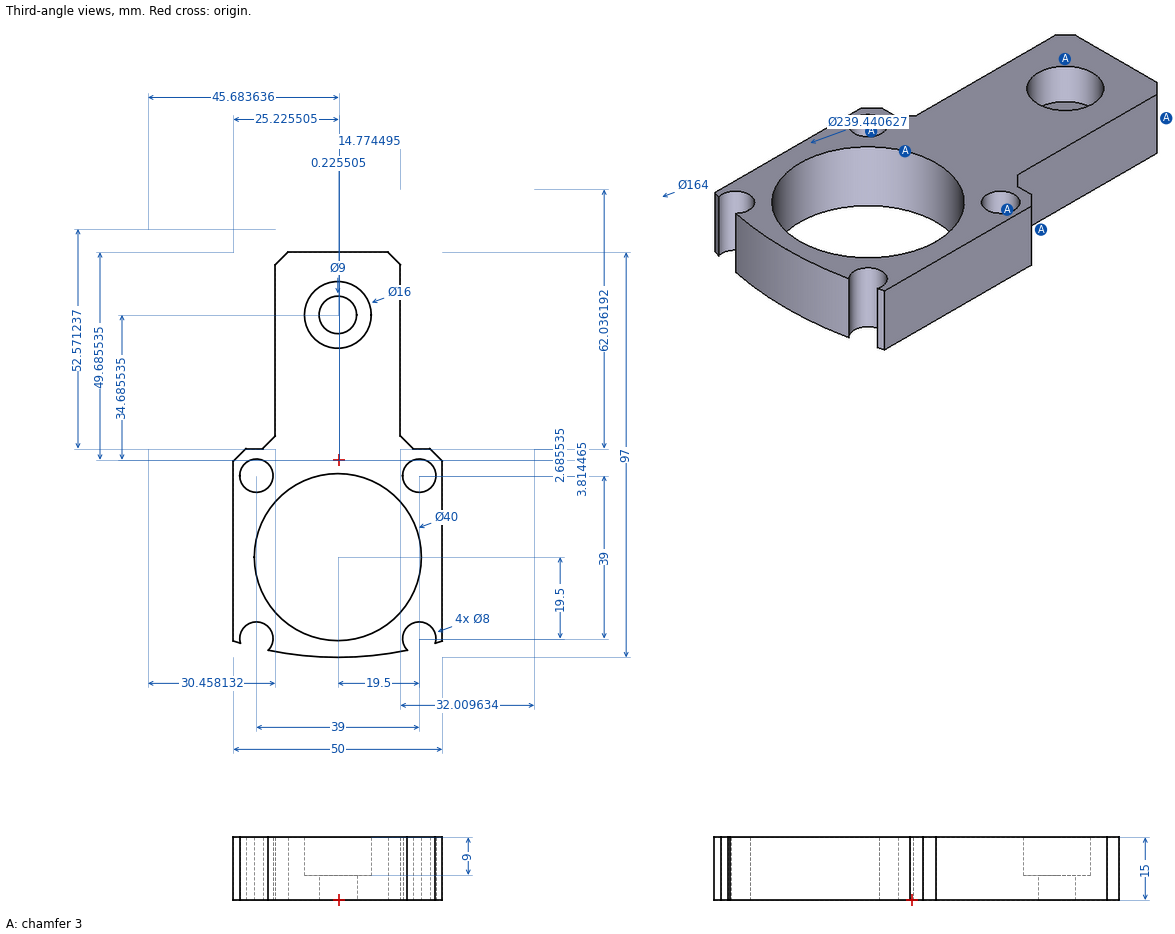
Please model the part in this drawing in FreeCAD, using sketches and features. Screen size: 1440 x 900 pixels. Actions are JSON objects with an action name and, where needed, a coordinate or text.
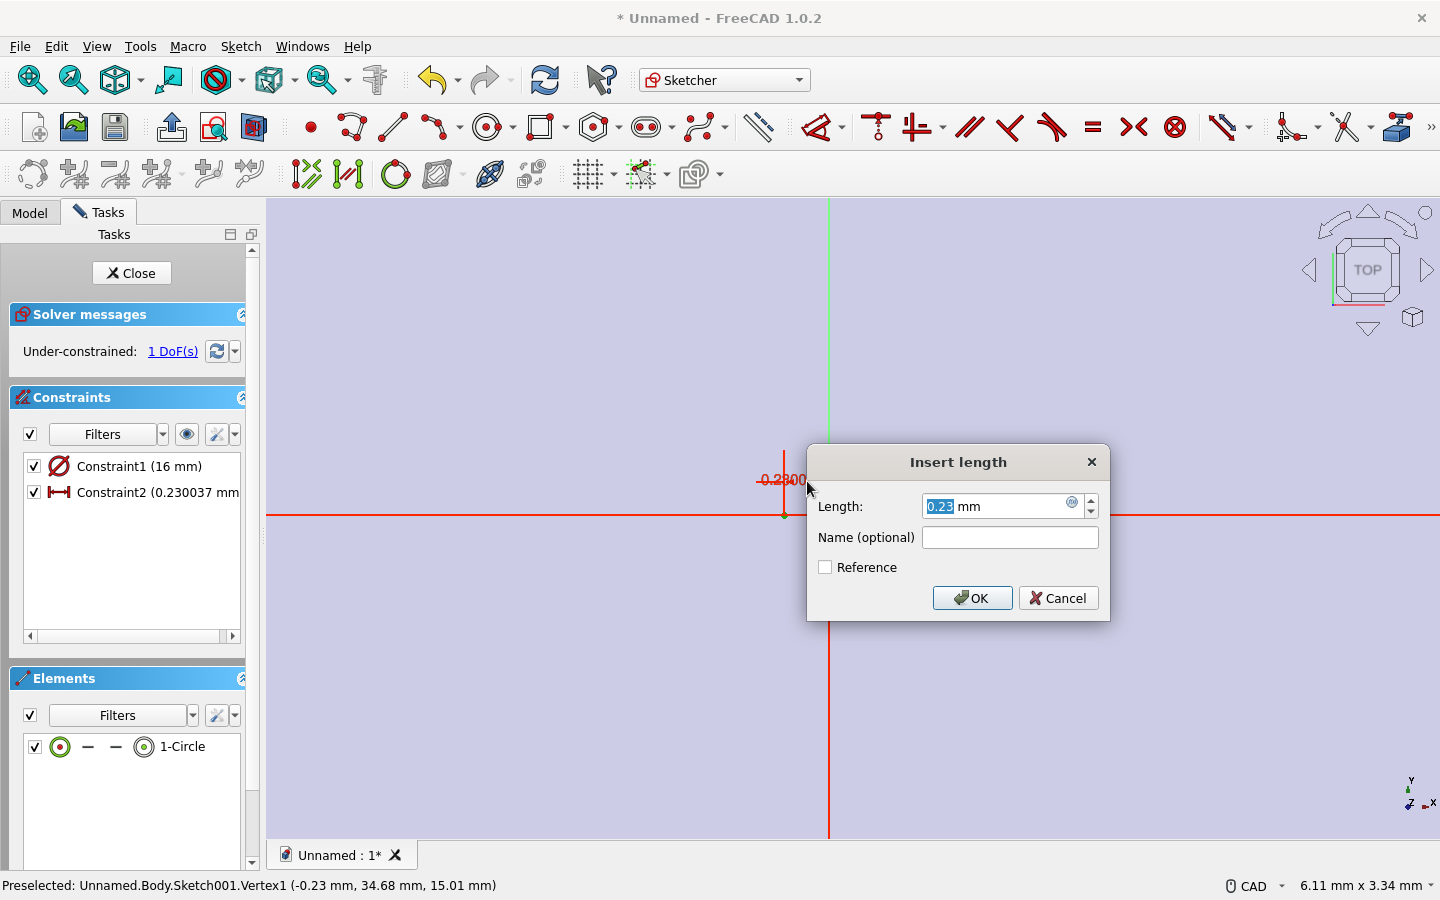
{"action": "type", "text": "0.225505"}
{"action": "key", "text": "Return"}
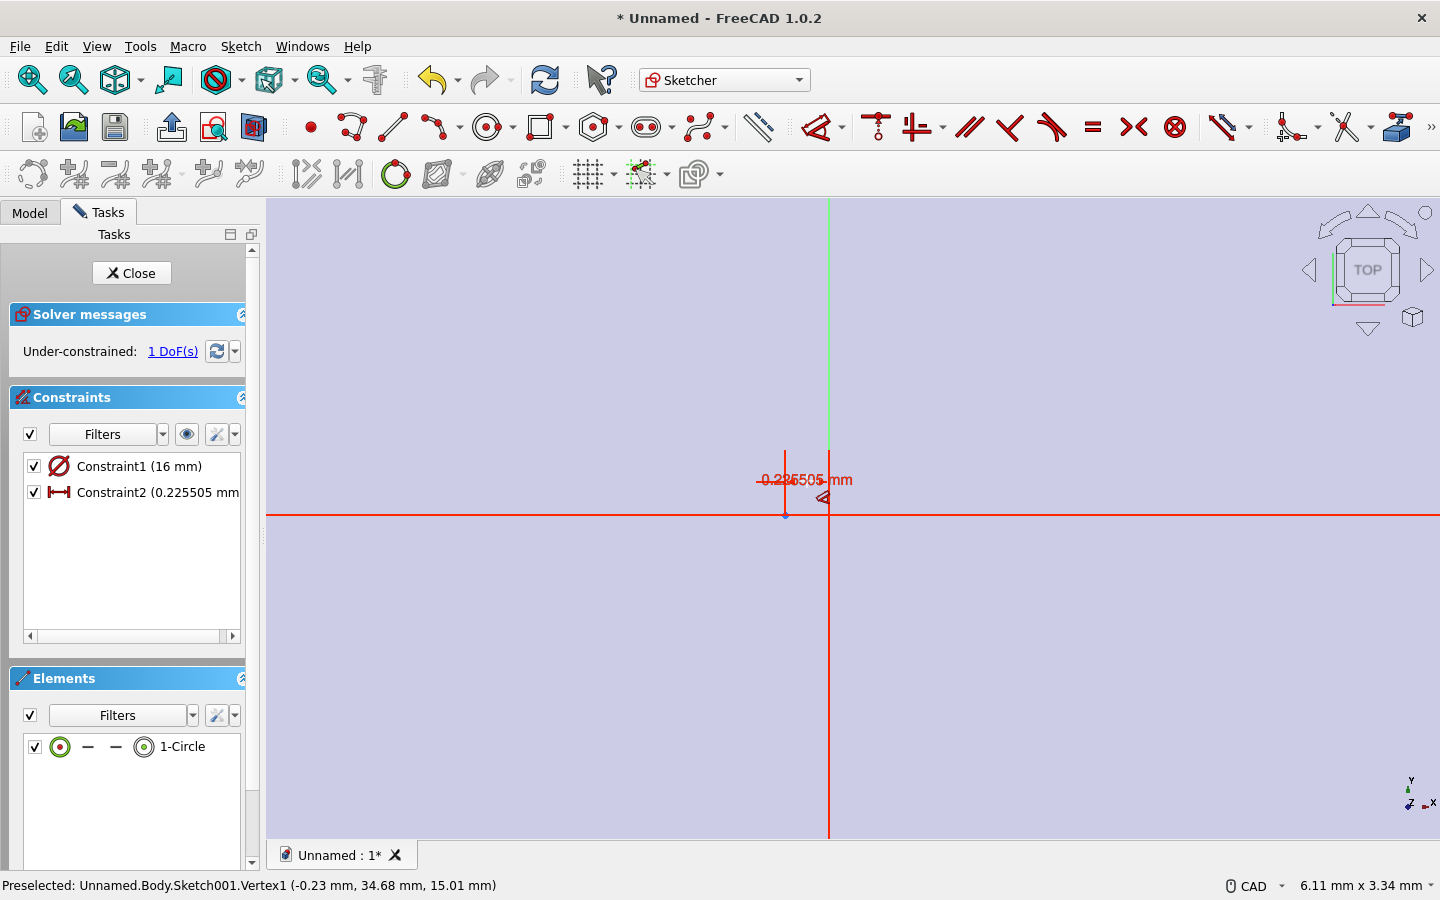
{"action": "scroll", "coordinate": [784, 519], "scroll_direction": "down", "scroll_amount": 10}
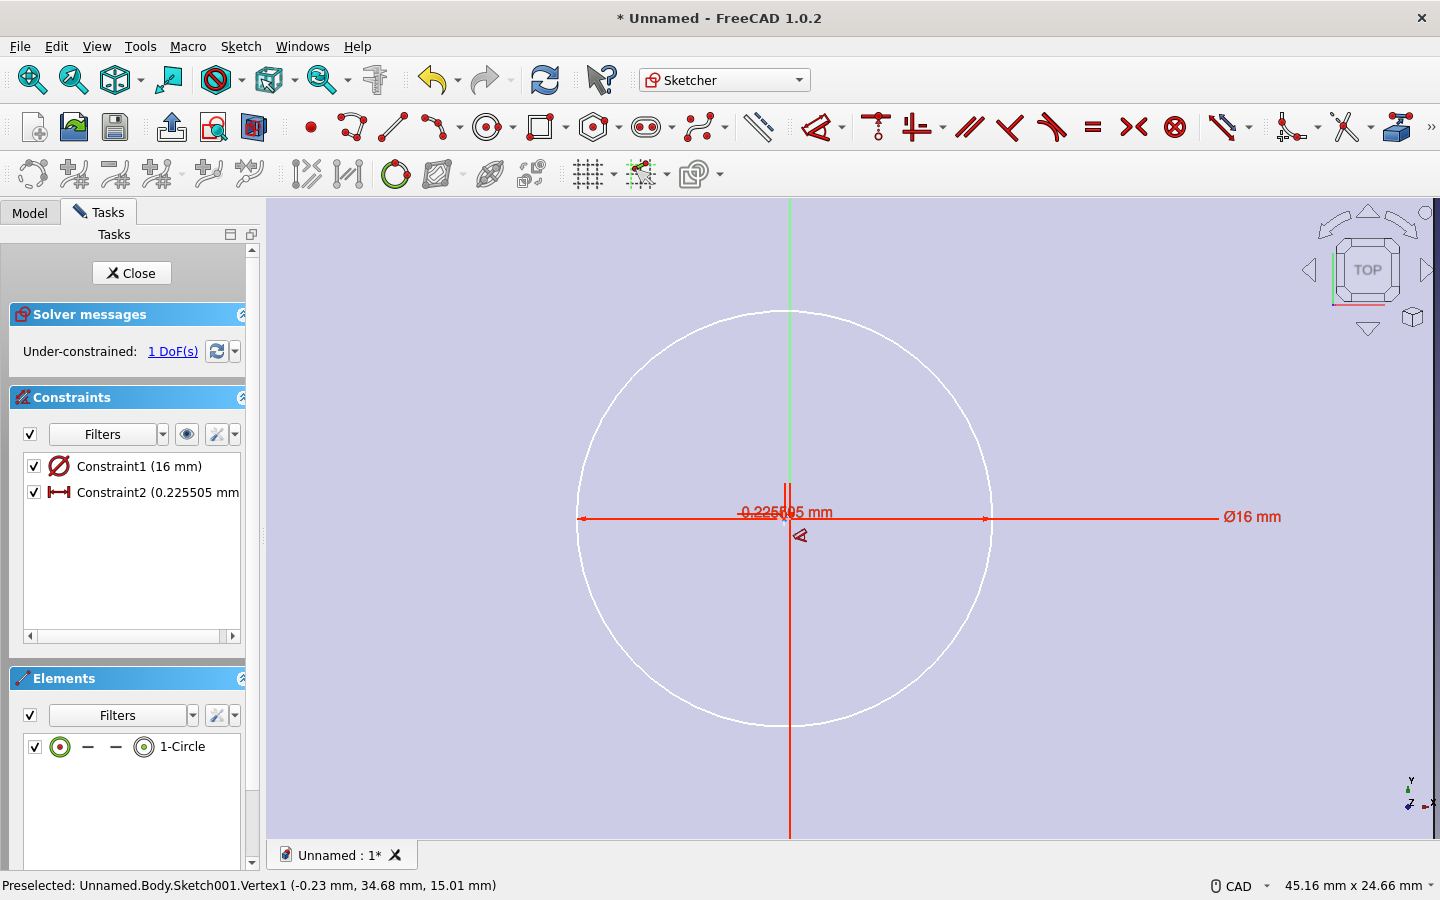
{"action": "left_click", "coordinate": [785, 519]}
{"action": "left_click", "coordinate": [824, 665]}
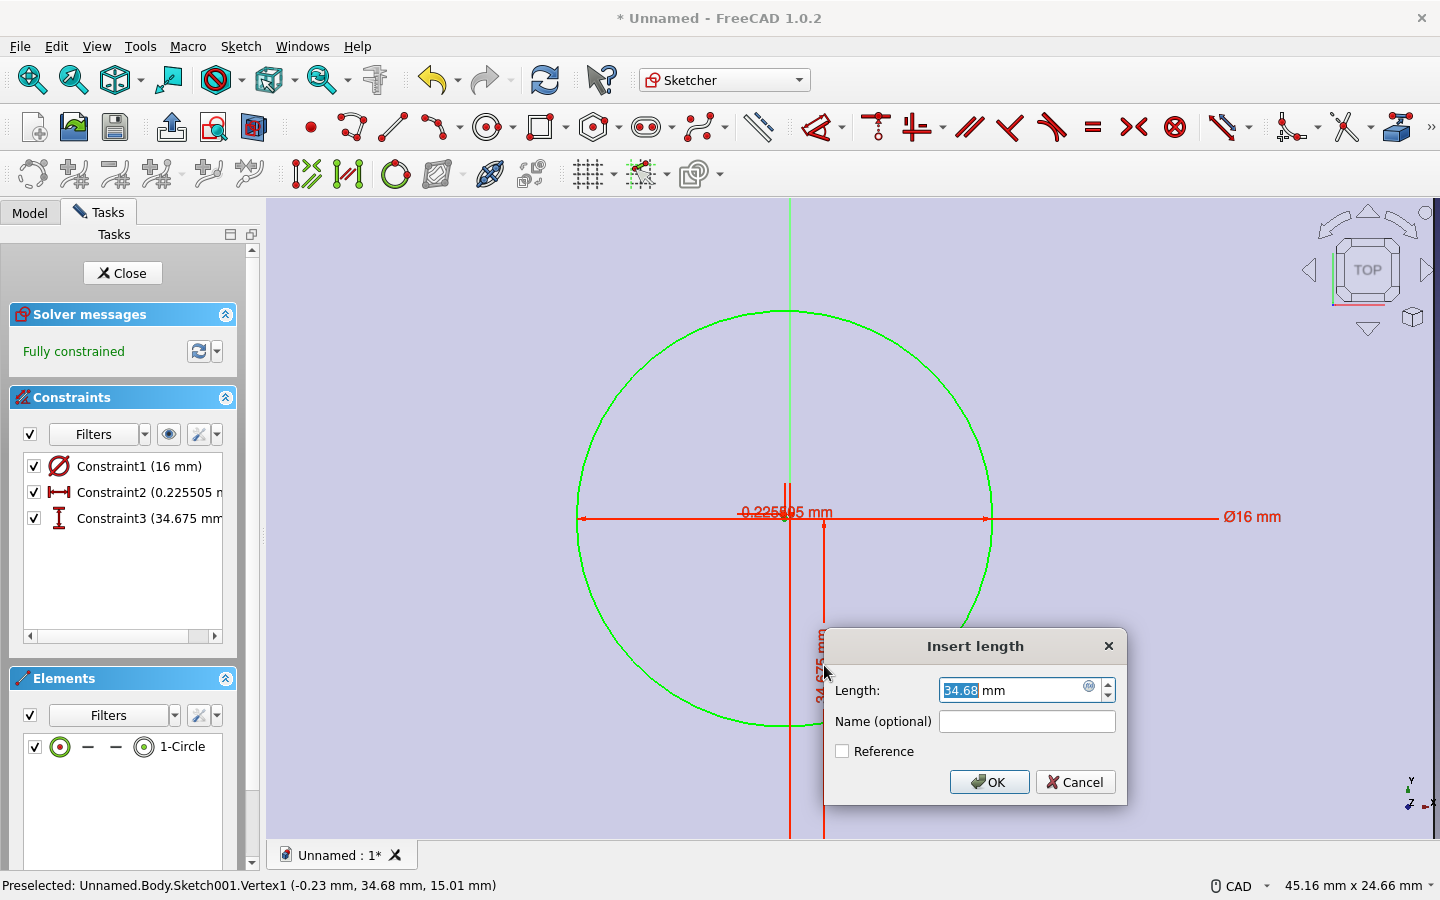
{"action": "type", "text": "34.685535"}
{"action": "key", "text": "Return"}
{"action": "key", "text": "Escape"}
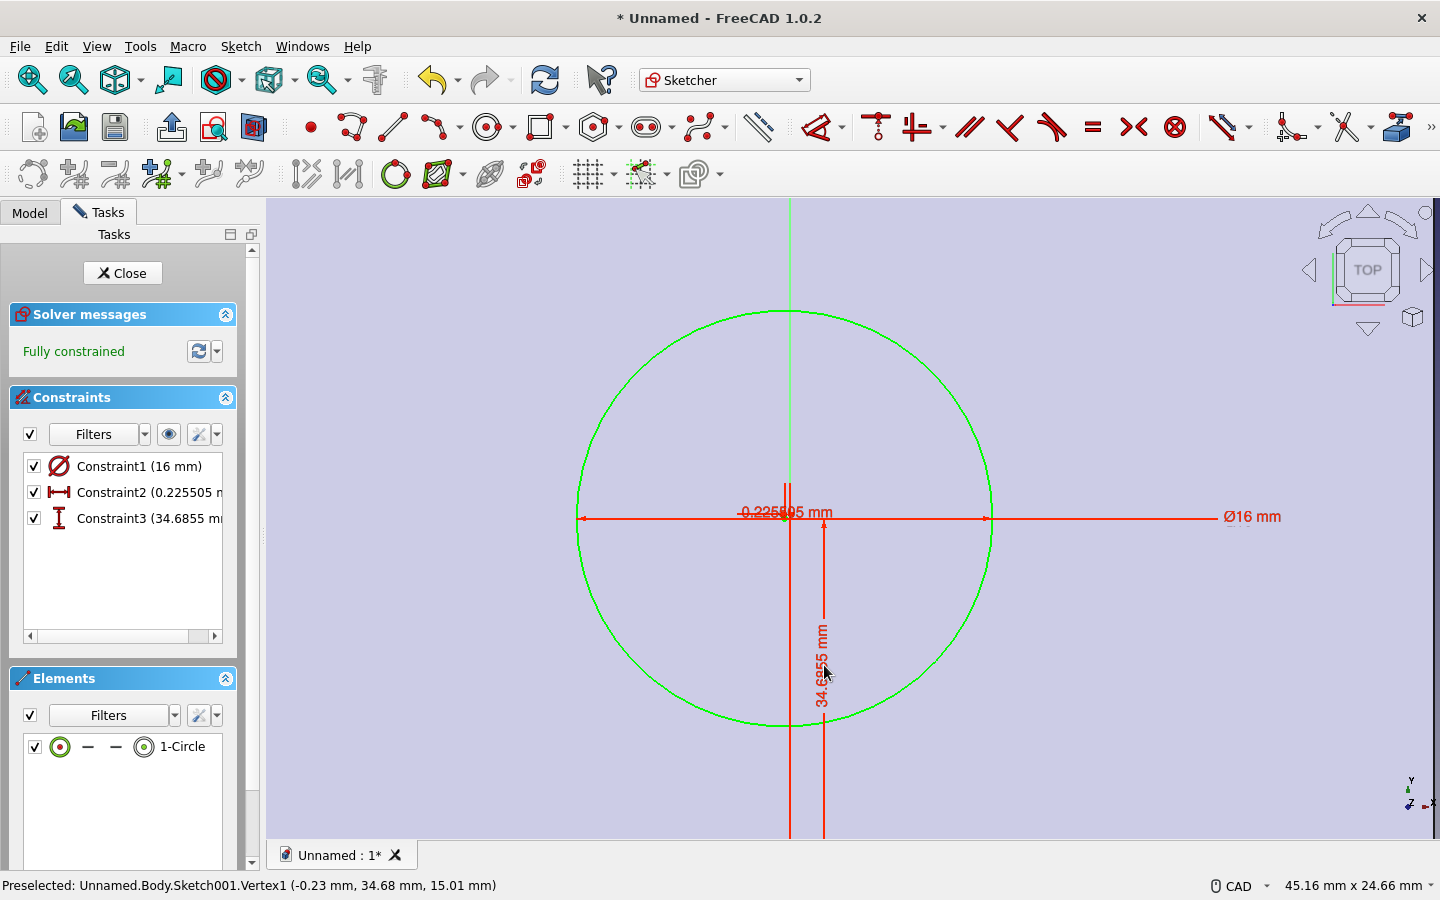
{"action": "left_click", "coordinate": [123, 273]}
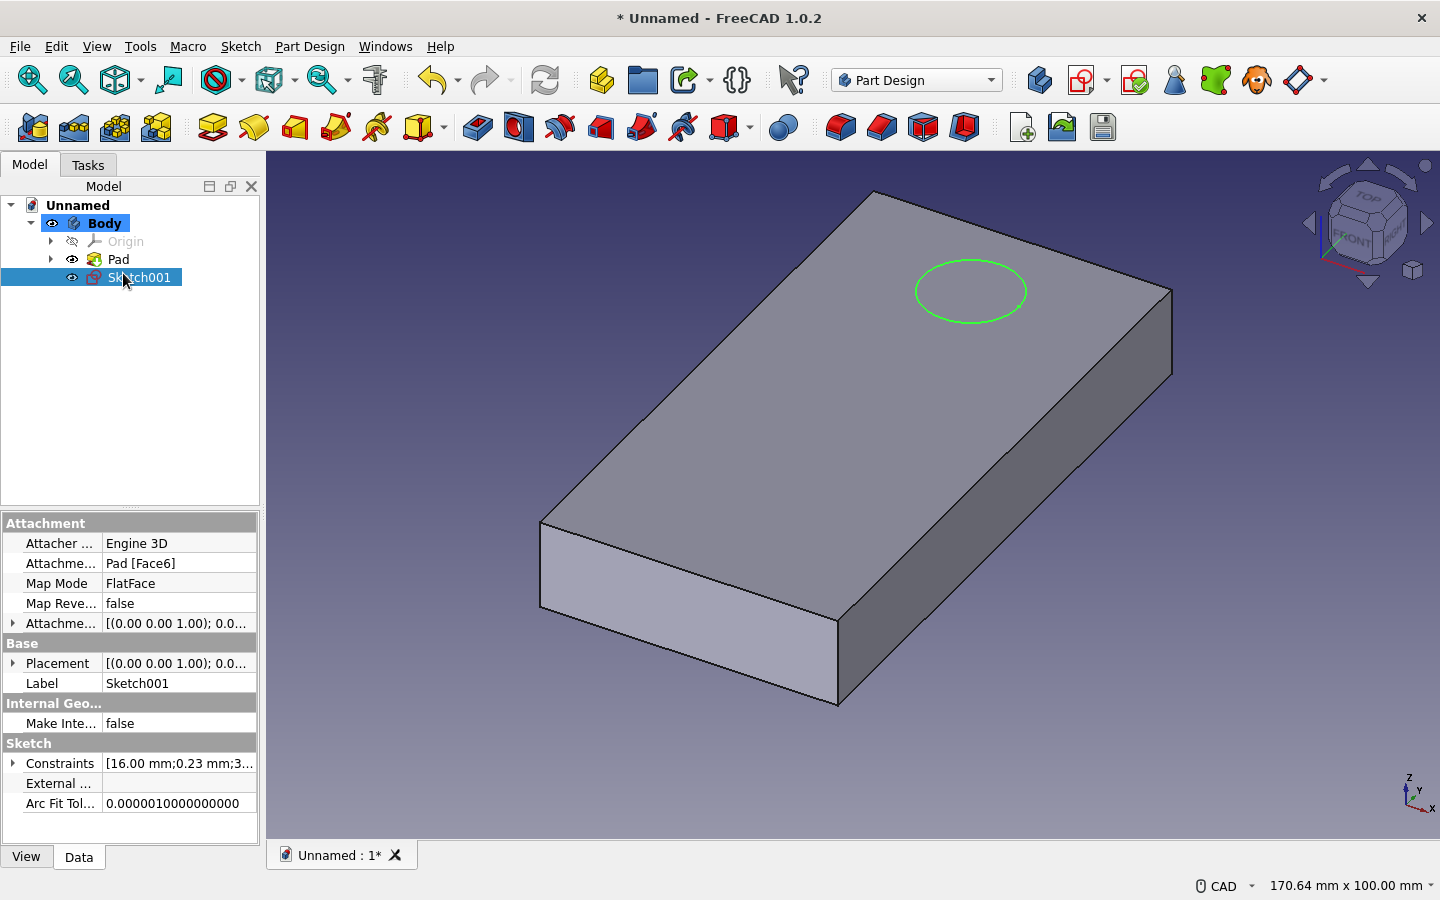
{"action": "left_click", "coordinate": [478, 128]}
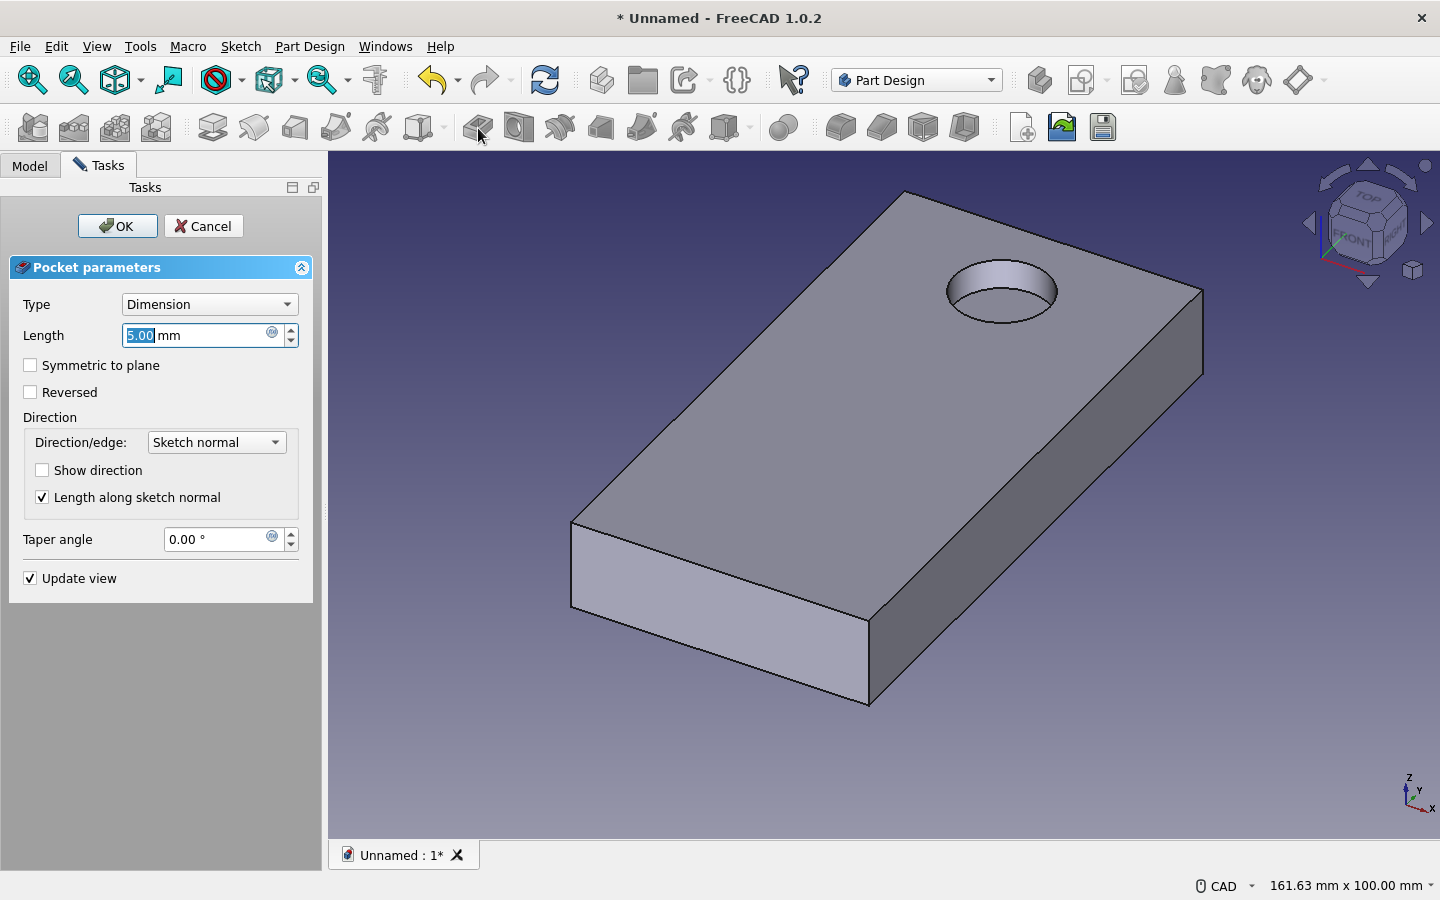
{"action": "type", "text": "9"}
{"action": "key", "text": "Tab"}